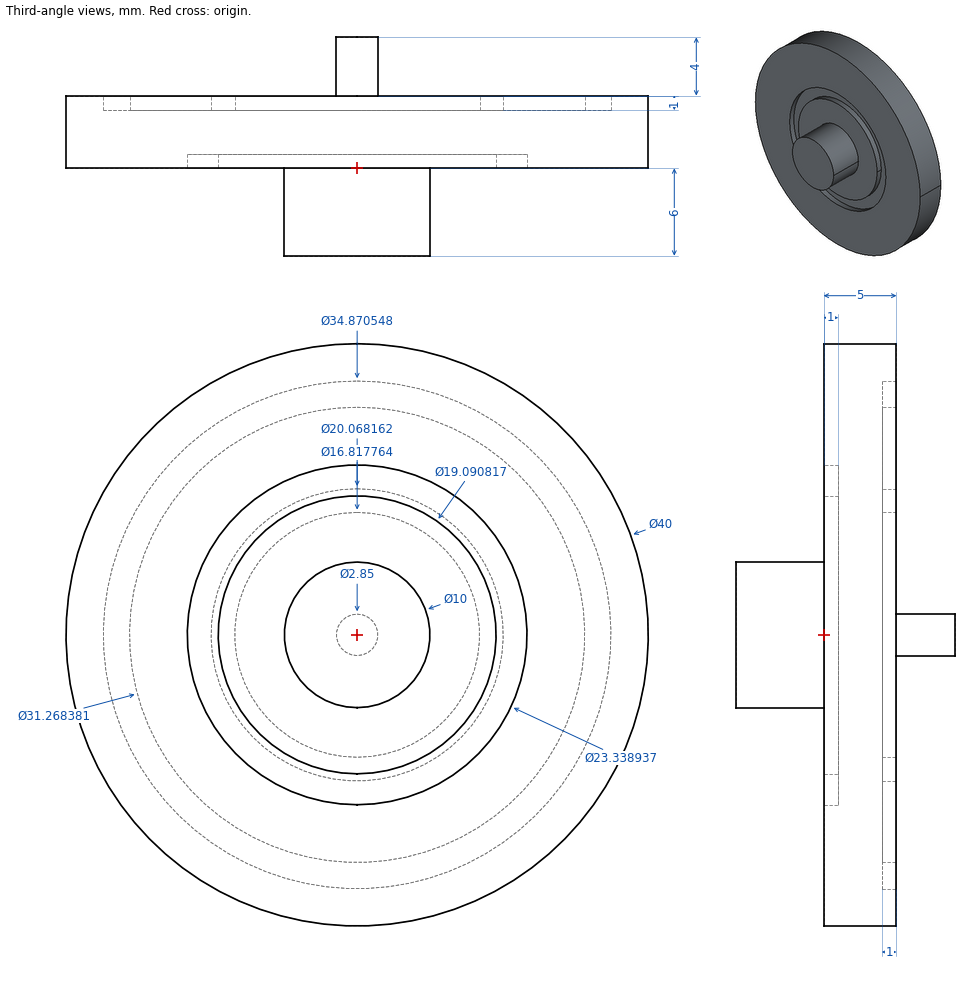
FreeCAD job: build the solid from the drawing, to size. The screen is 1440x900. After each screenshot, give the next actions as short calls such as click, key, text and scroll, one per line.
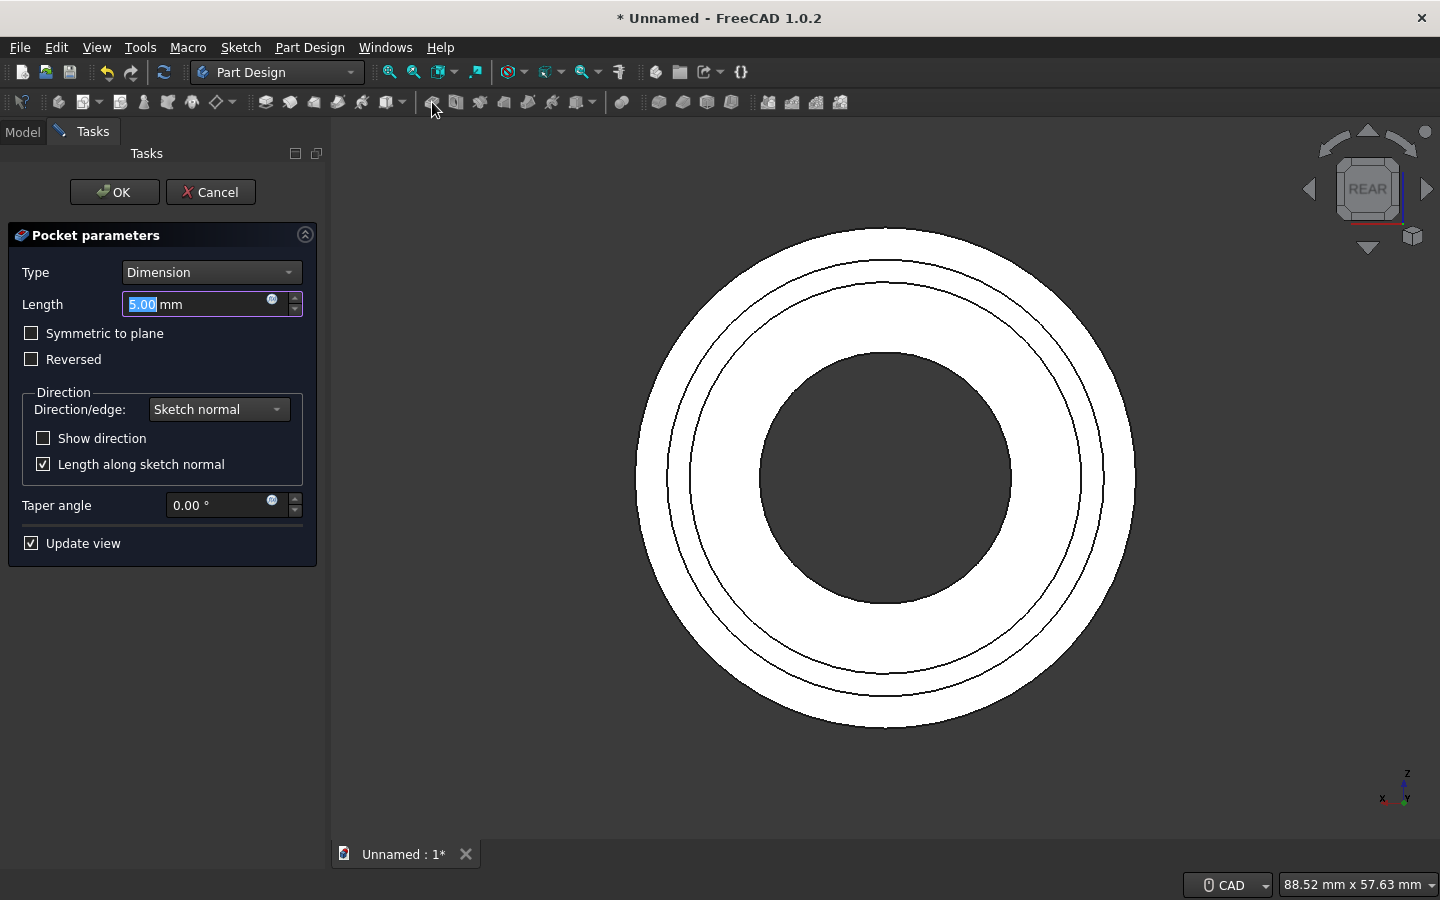
text(1)
key(Tab)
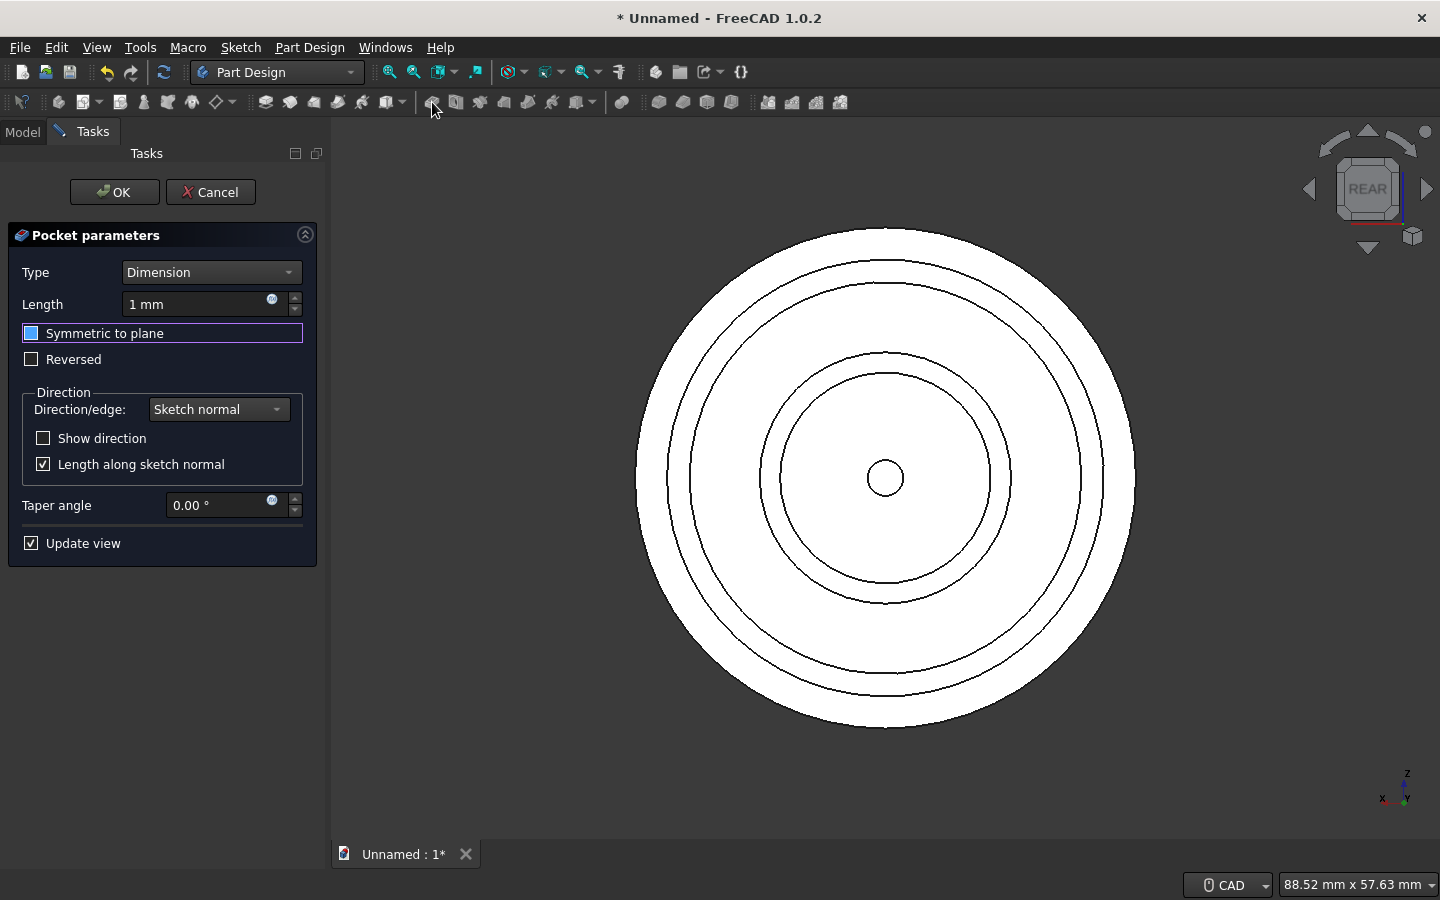
click(115, 192)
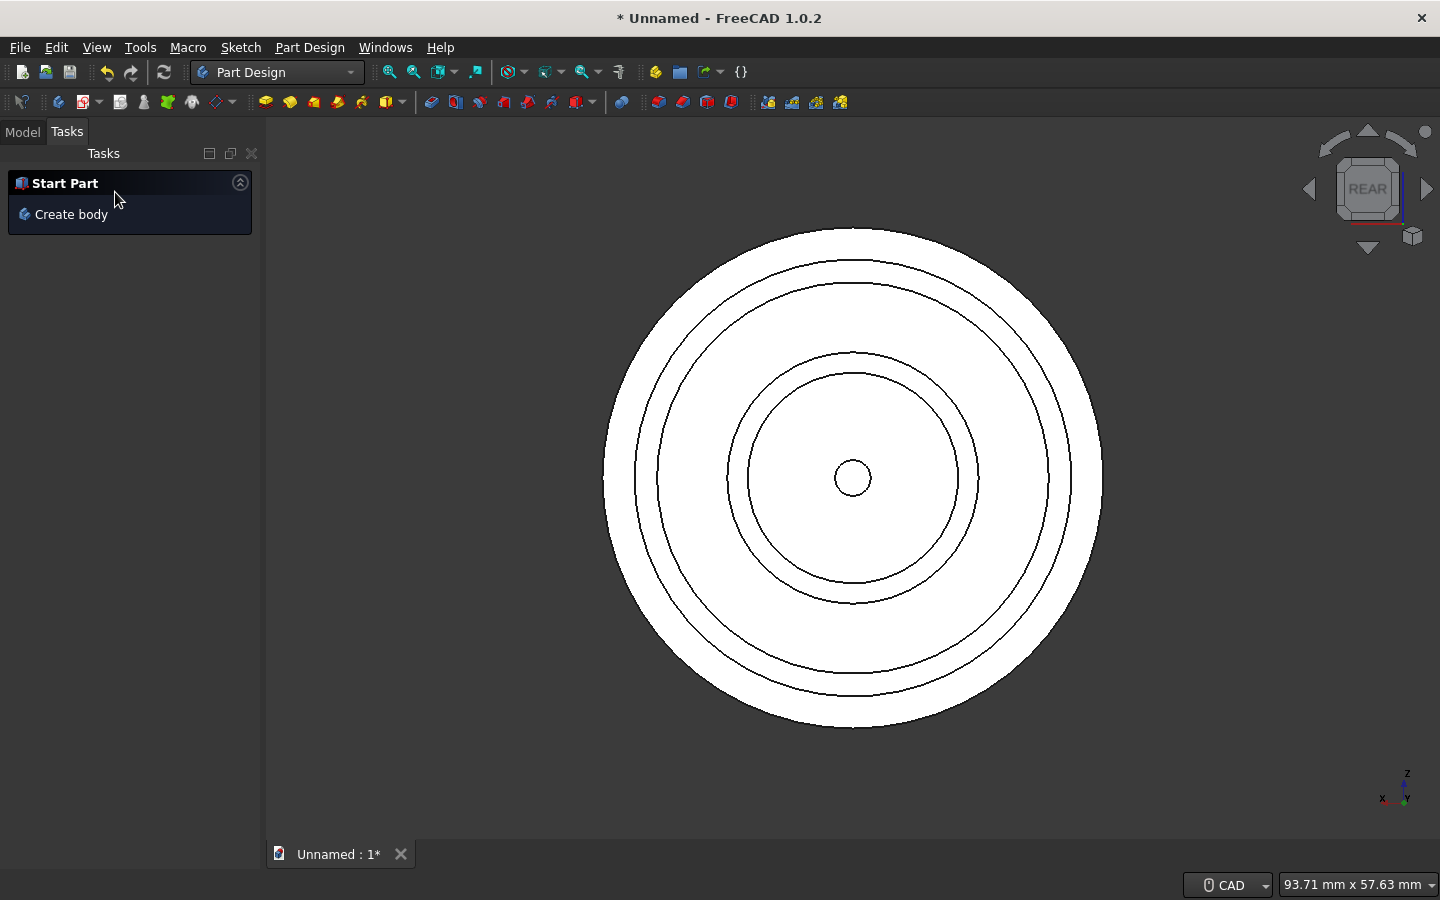
key(0)